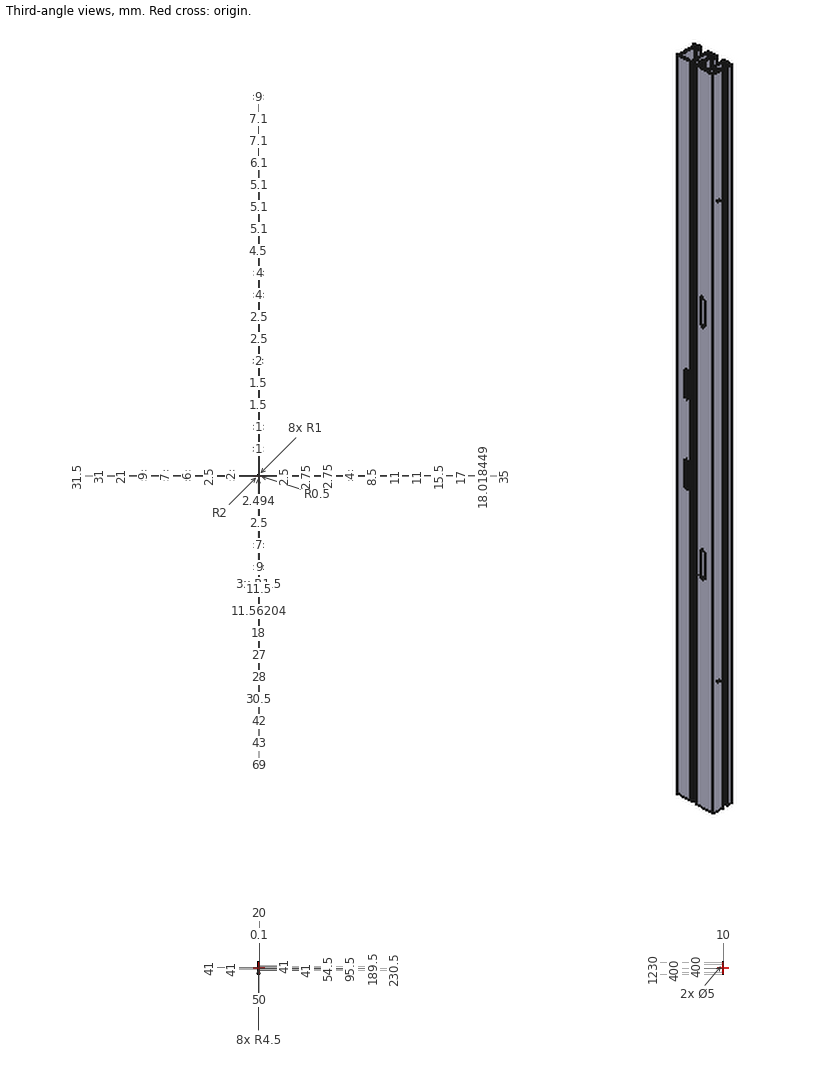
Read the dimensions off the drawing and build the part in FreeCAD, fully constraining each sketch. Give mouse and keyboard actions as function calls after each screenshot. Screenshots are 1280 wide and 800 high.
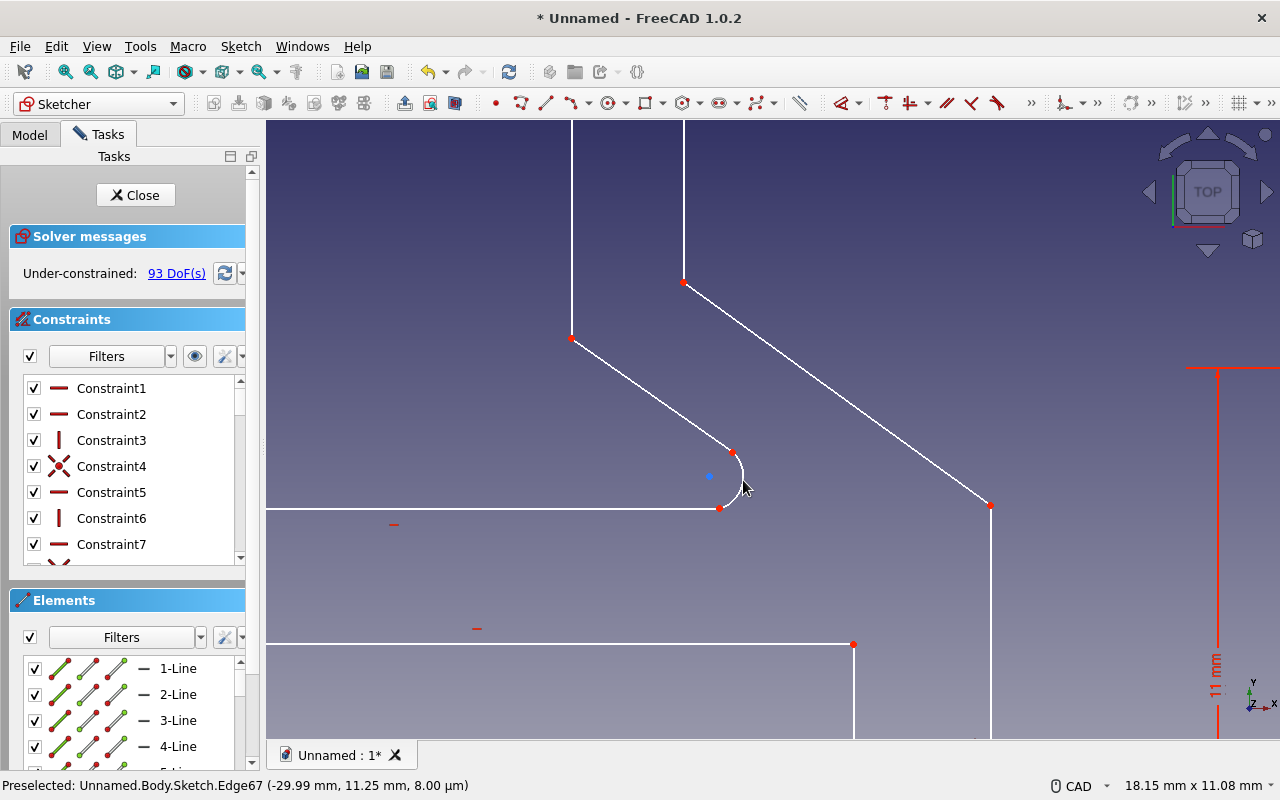
scroll(742, 475, down, 10)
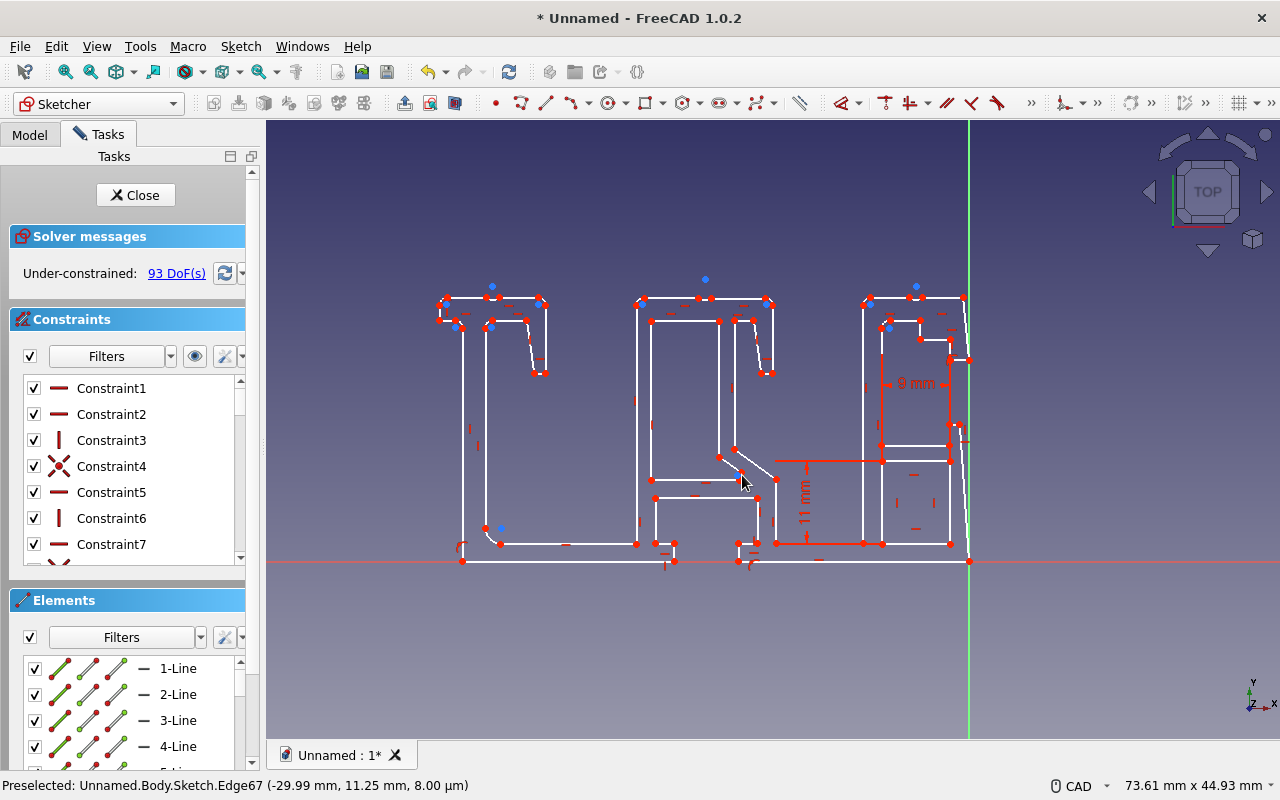
click(728, 299)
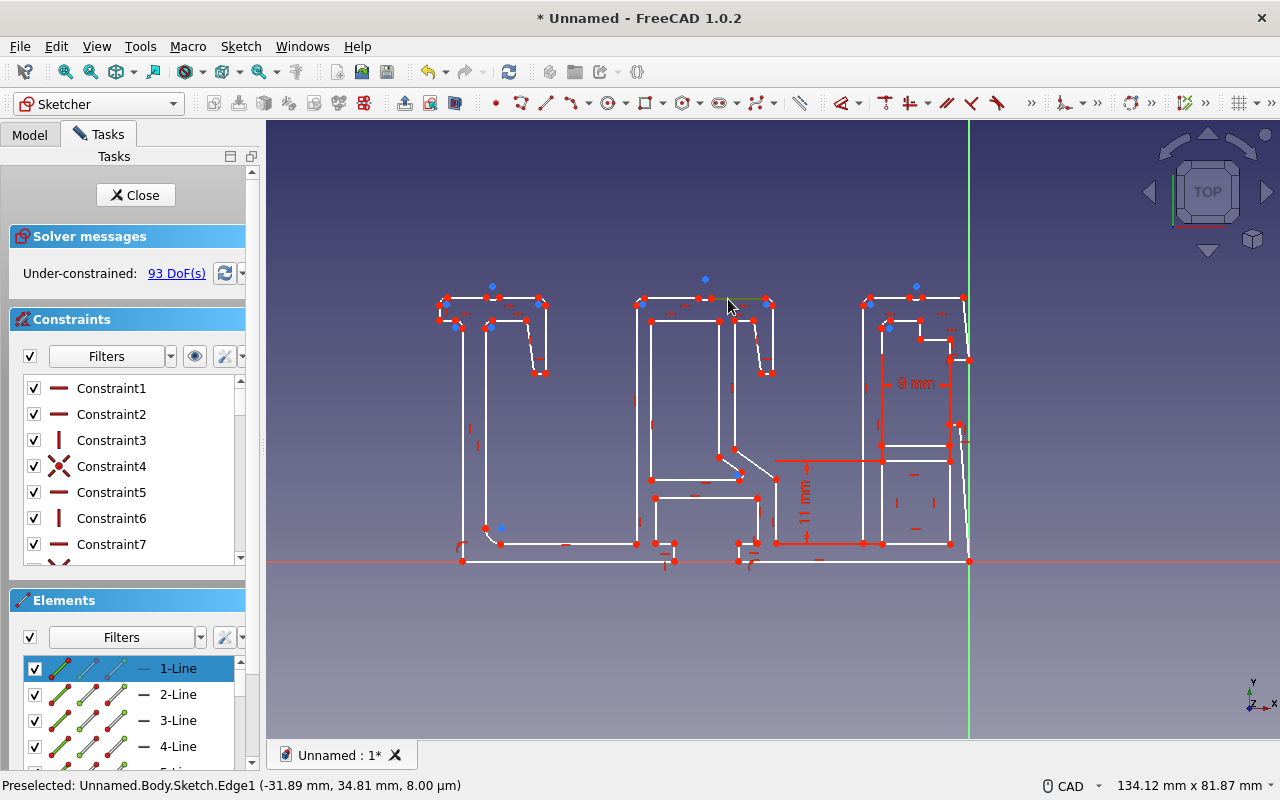
scroll(771, 300, up, 5)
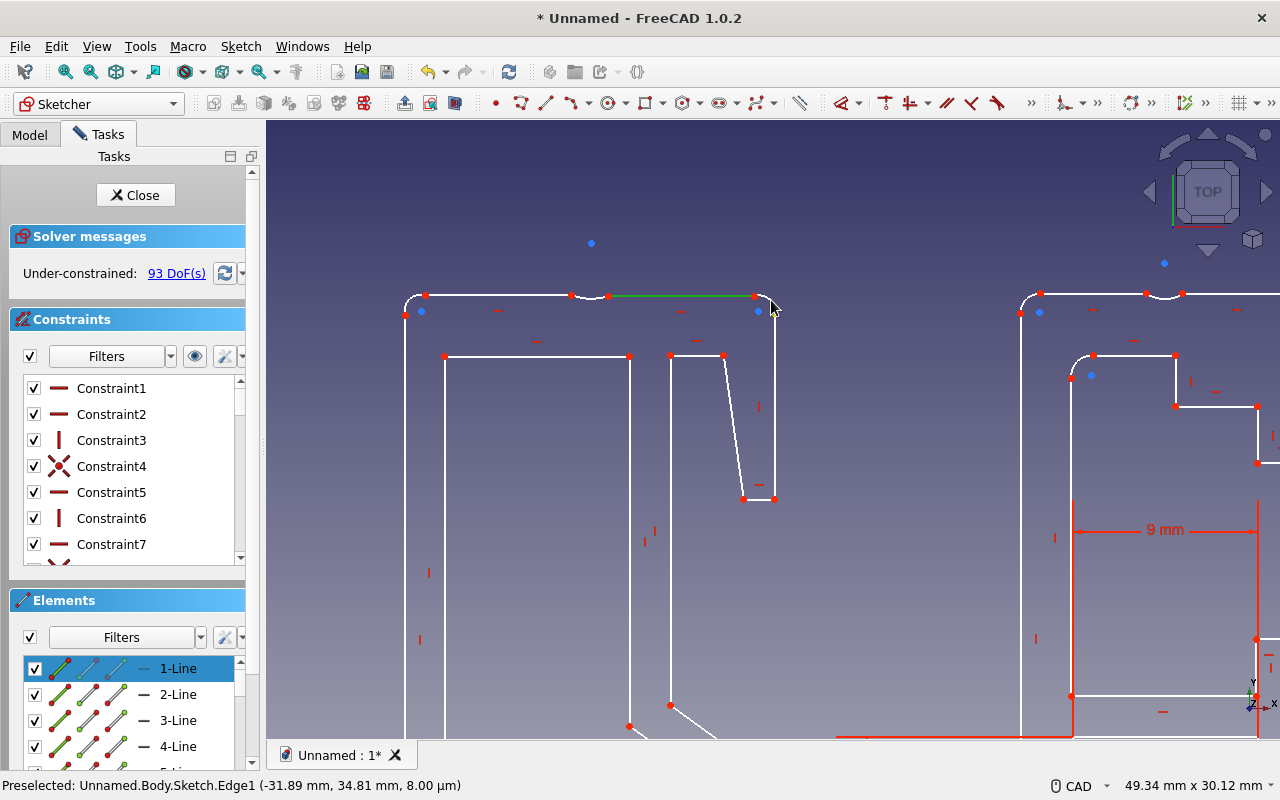
click(769, 299)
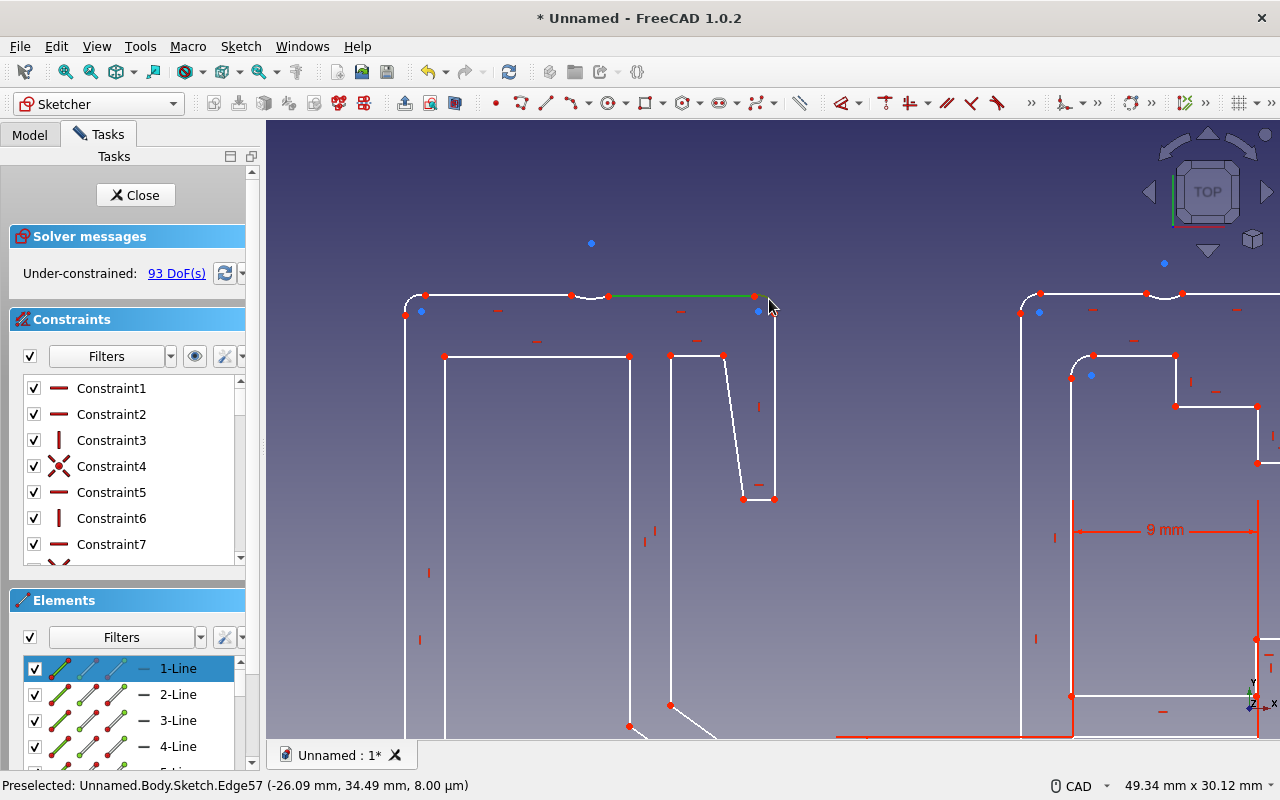
click(997, 104)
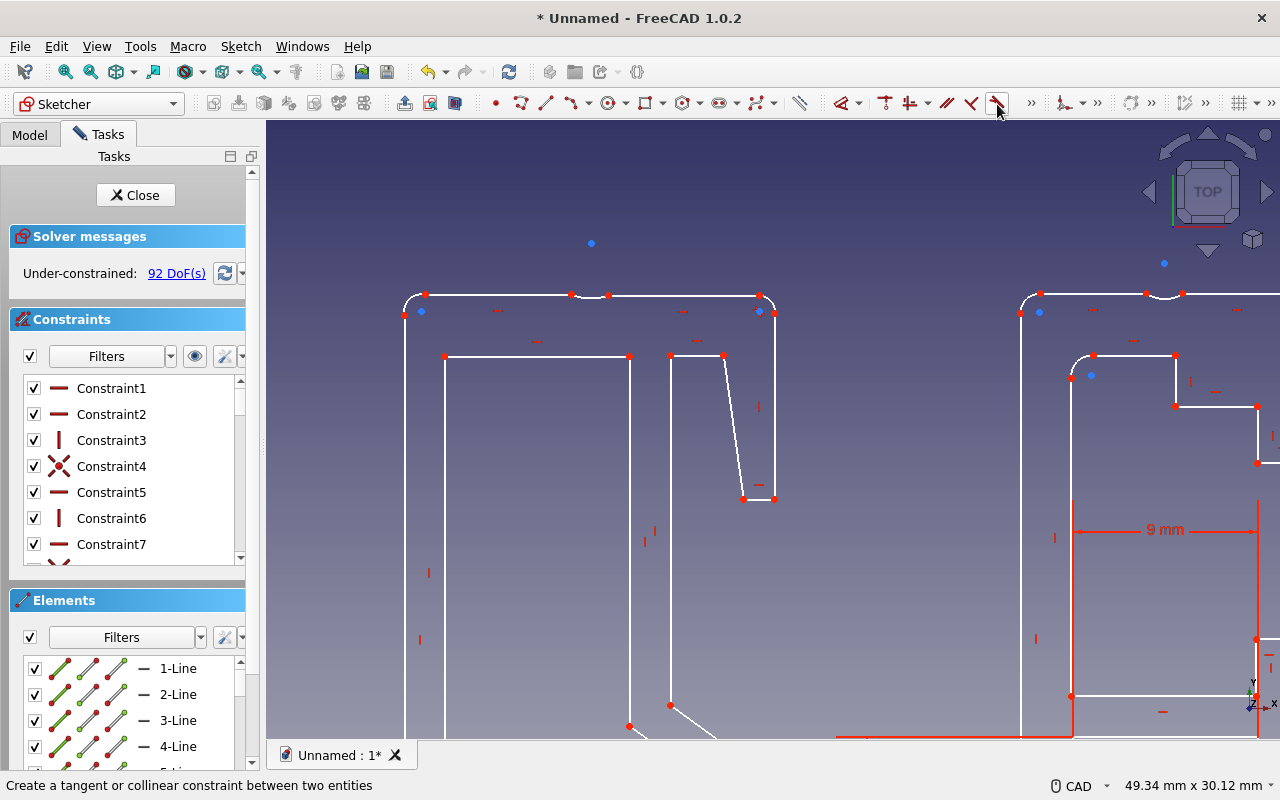
click(528, 295)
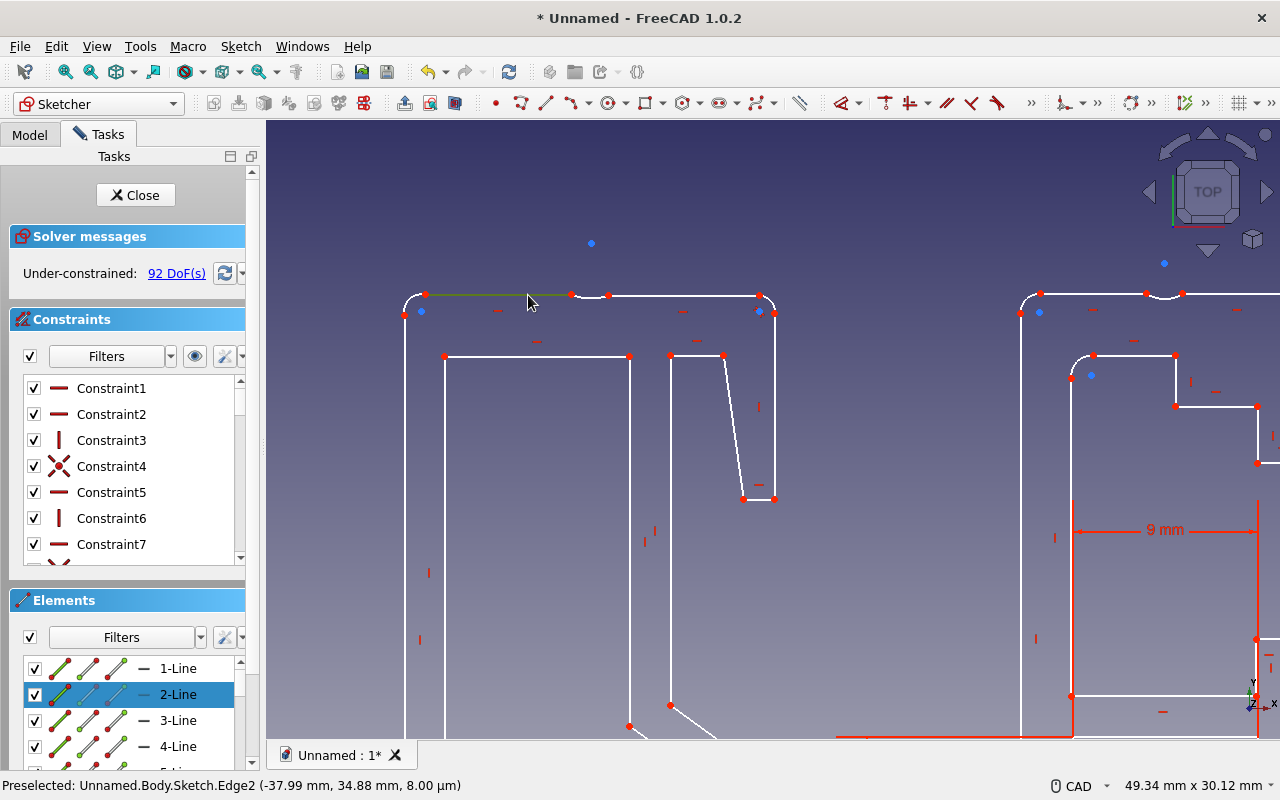
scroll(415, 295, up, 2)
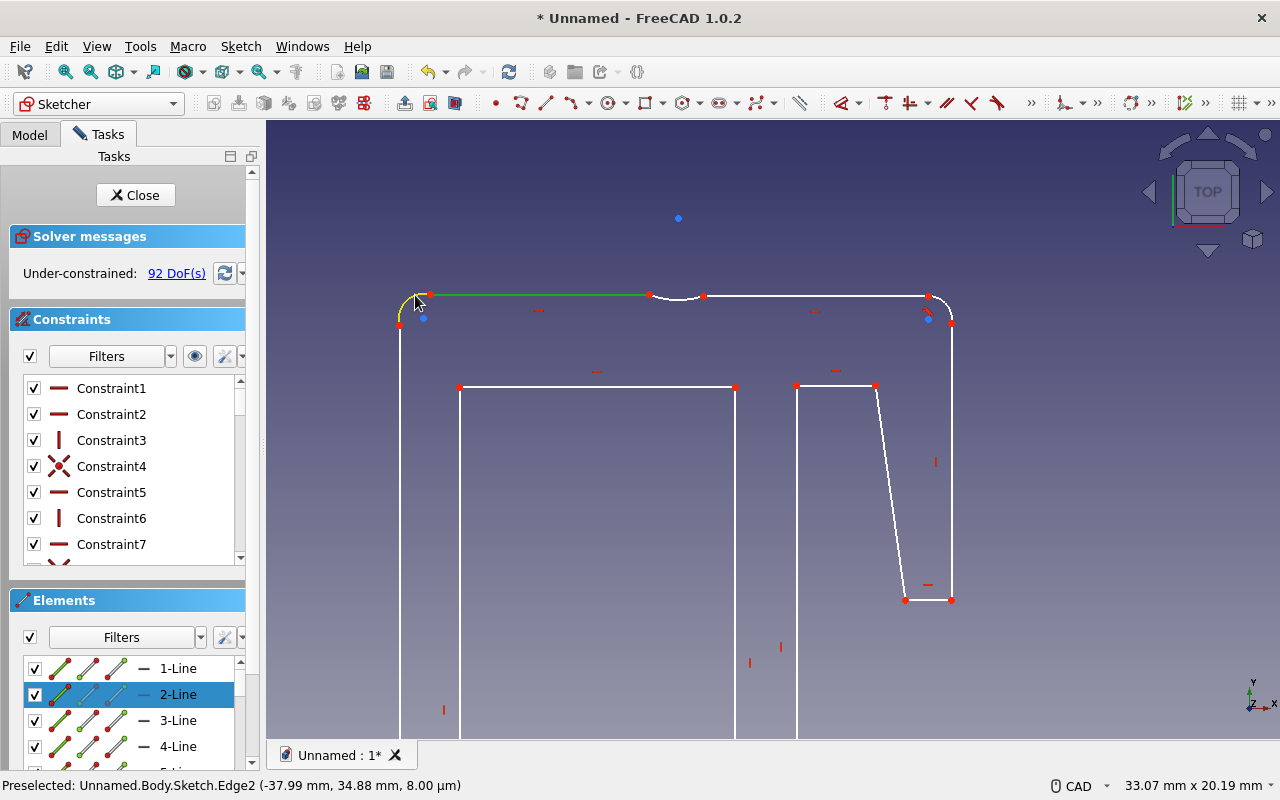
click(415, 296)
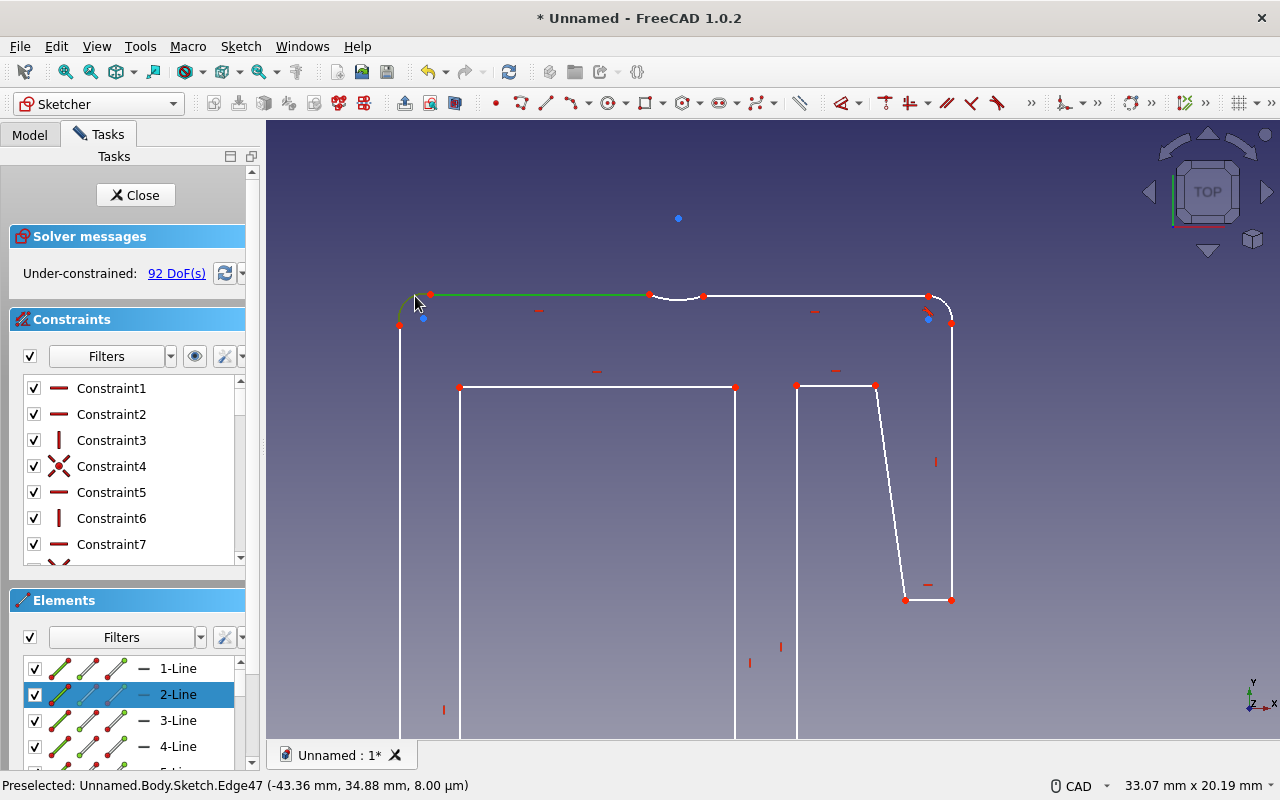
click(997, 104)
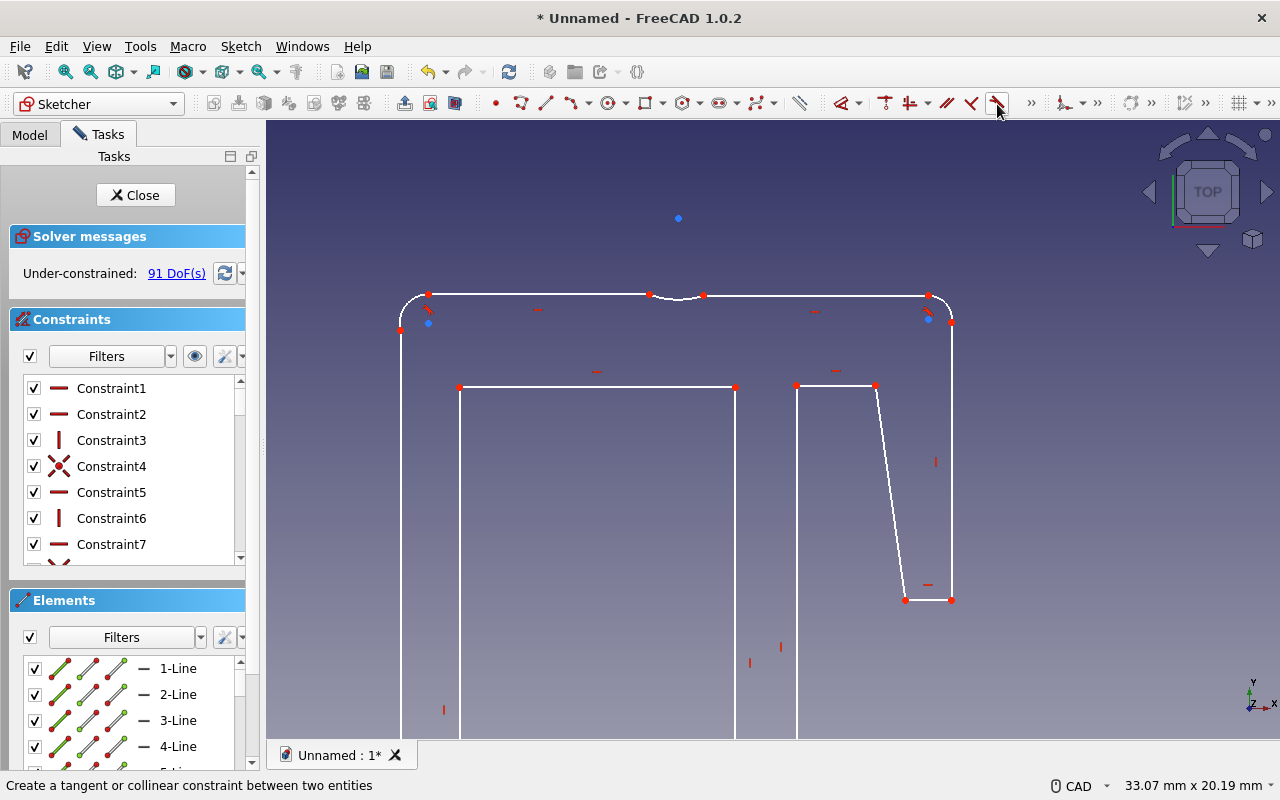
scroll(714, 299, down, 7)